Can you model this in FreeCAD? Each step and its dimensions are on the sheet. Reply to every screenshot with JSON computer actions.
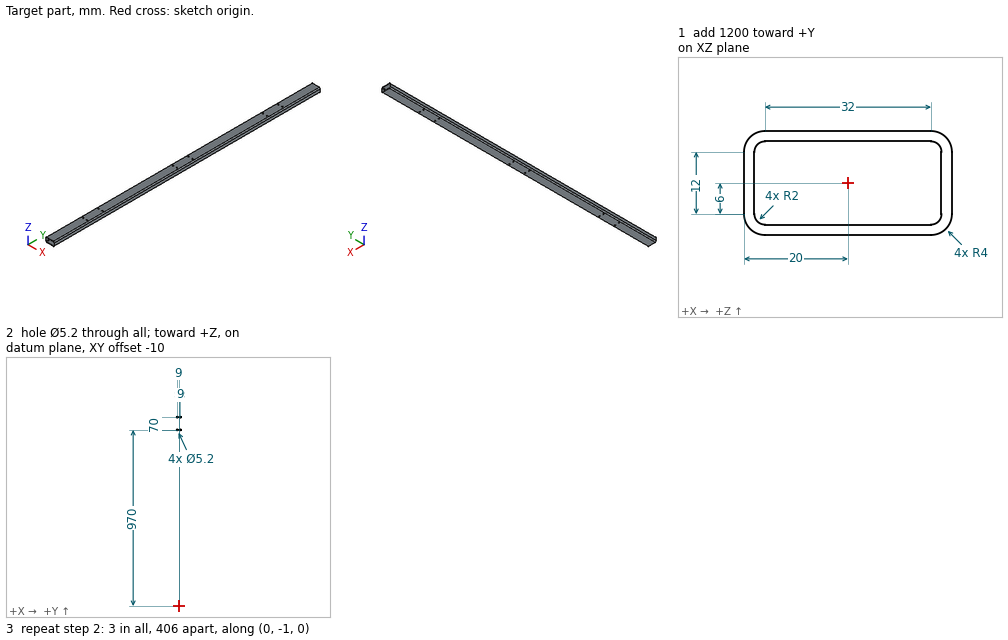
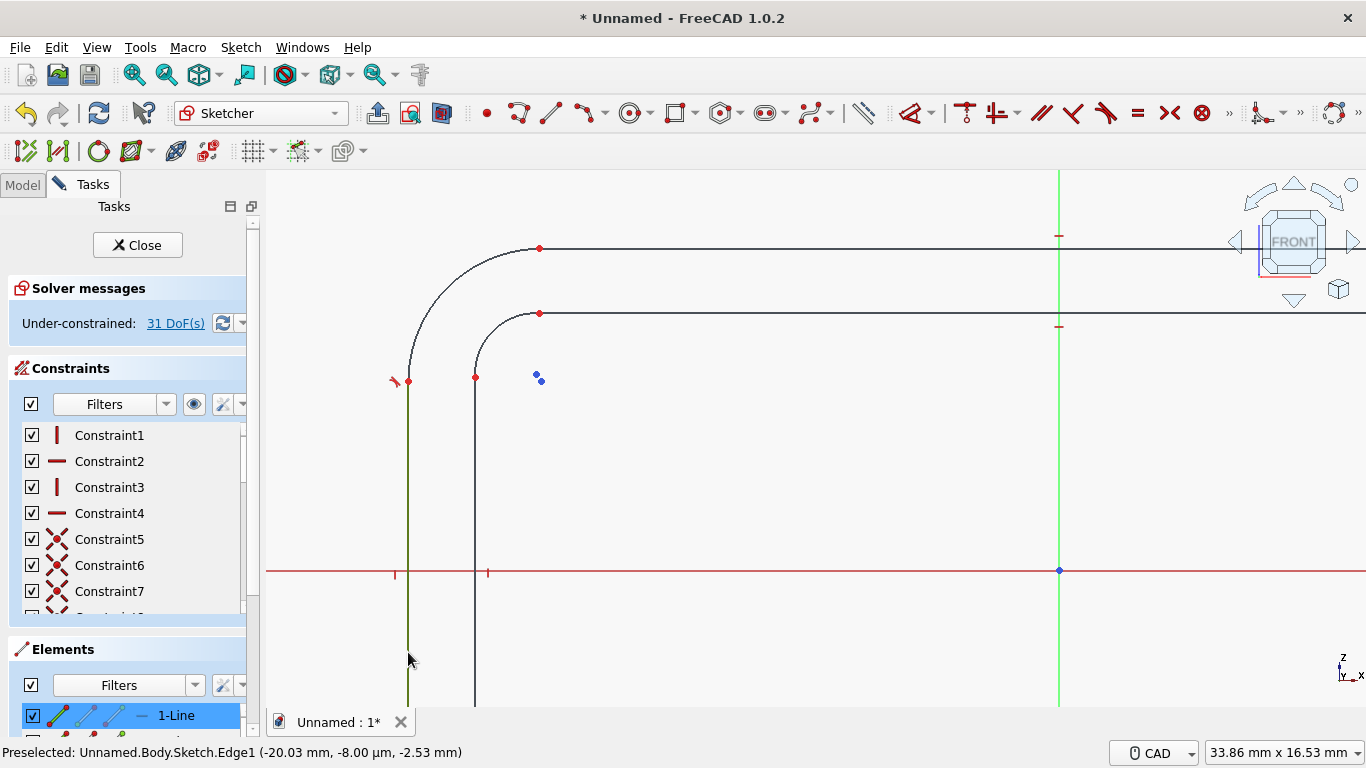
{"action": "scroll", "coordinate": [493, 330], "scroll_direction": "down", "scroll_amount": 4}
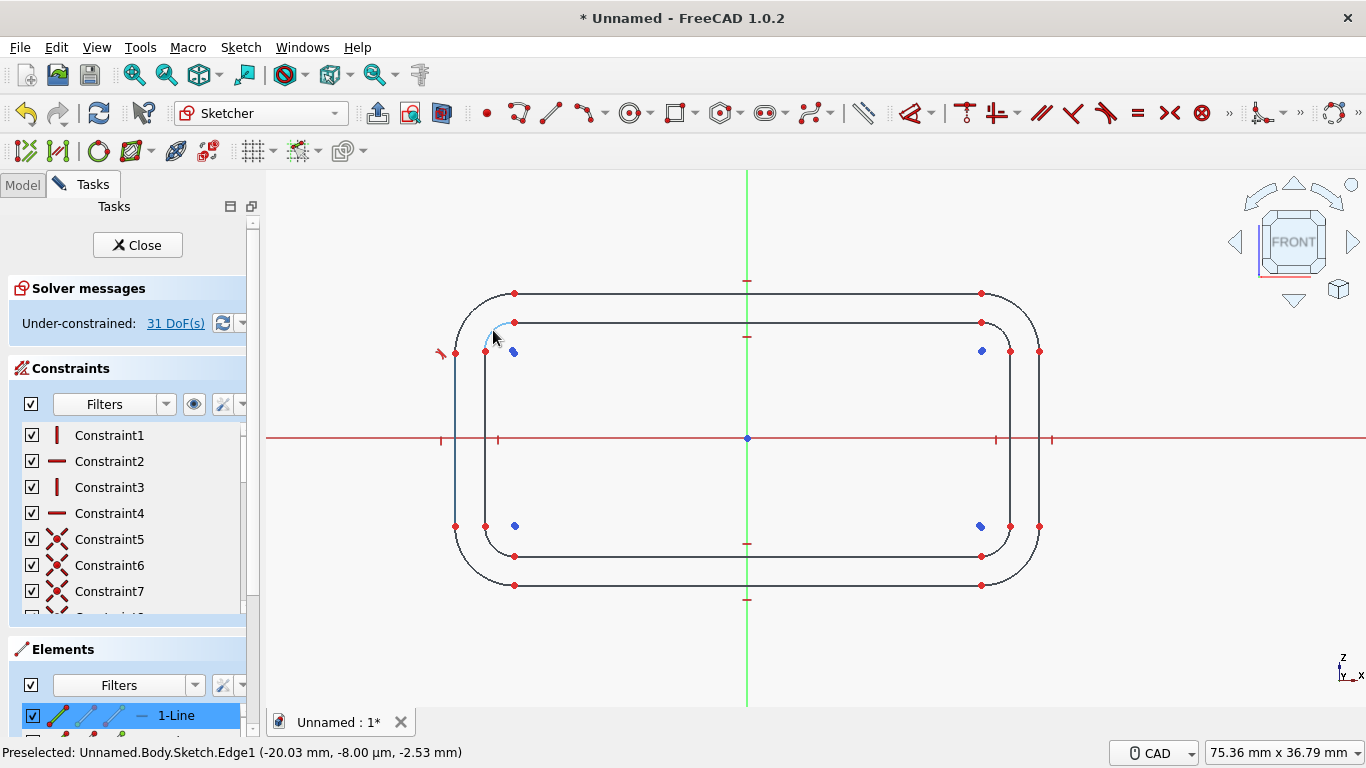
{"action": "left_click", "coordinate": [462, 553]}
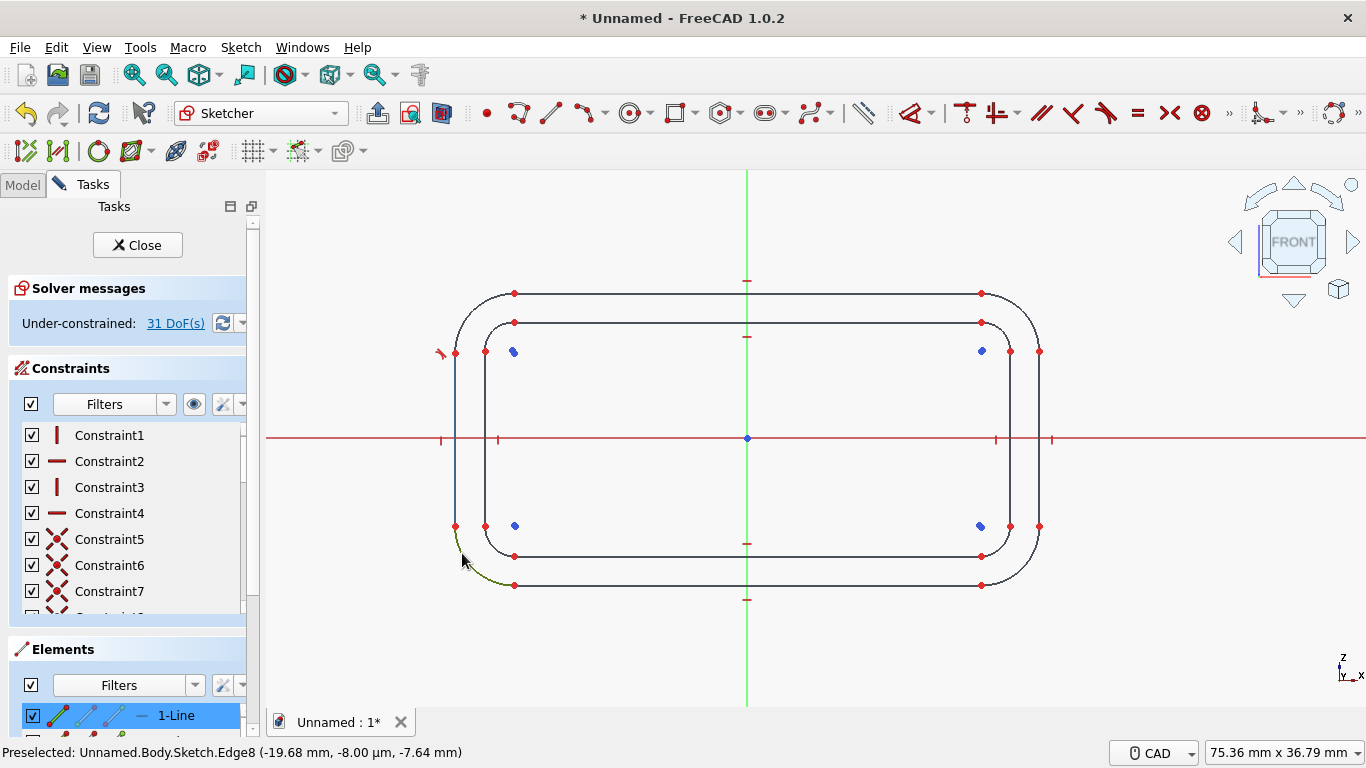
{"action": "left_click", "coordinate": [1106, 114]}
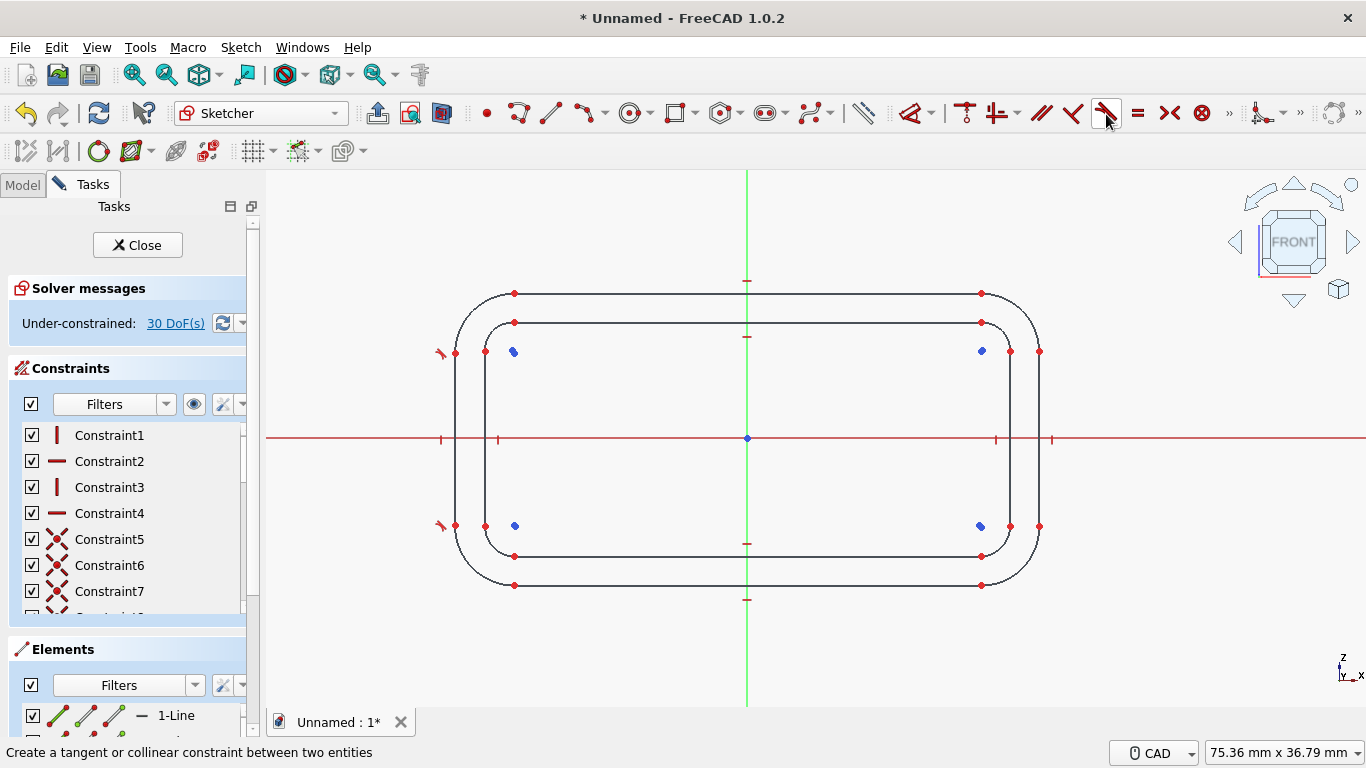
{"action": "left_click", "coordinate": [654, 294]}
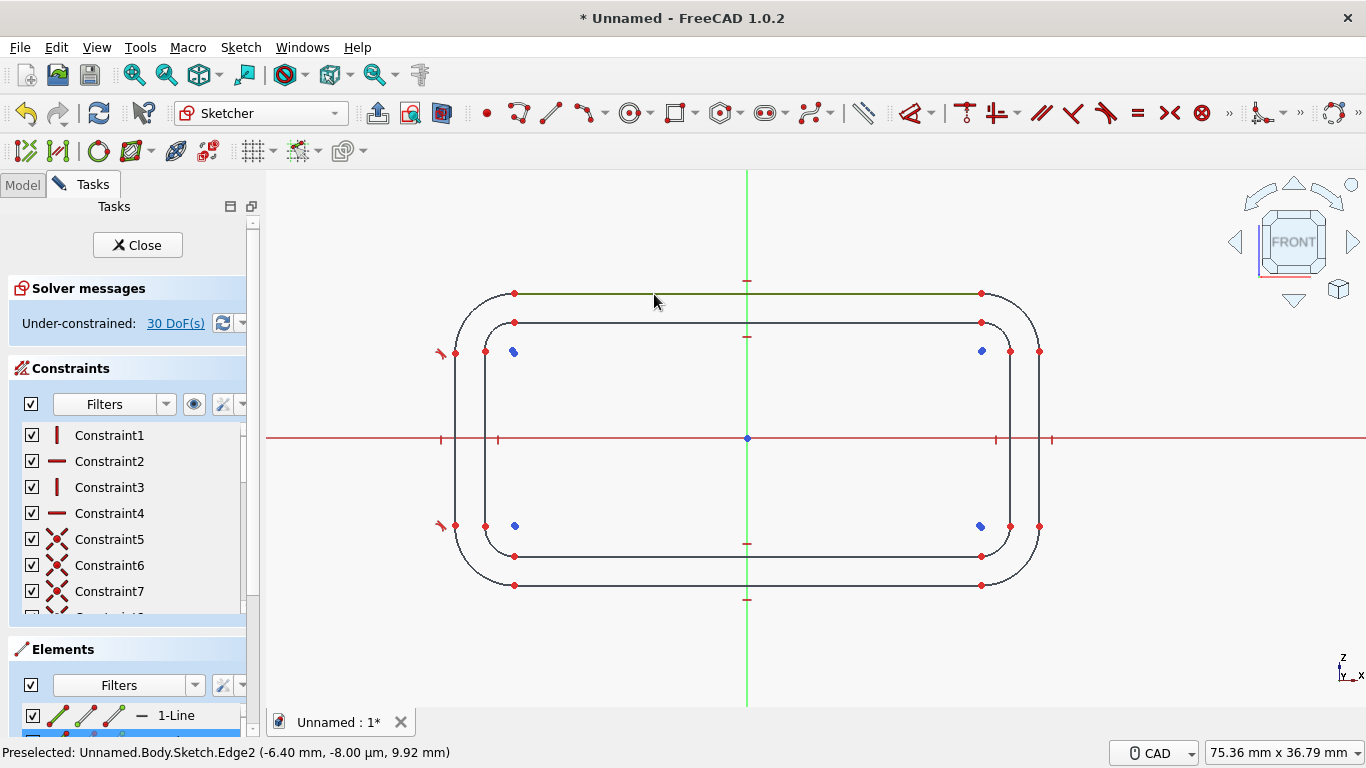
{"action": "left_click", "coordinate": [487, 300]}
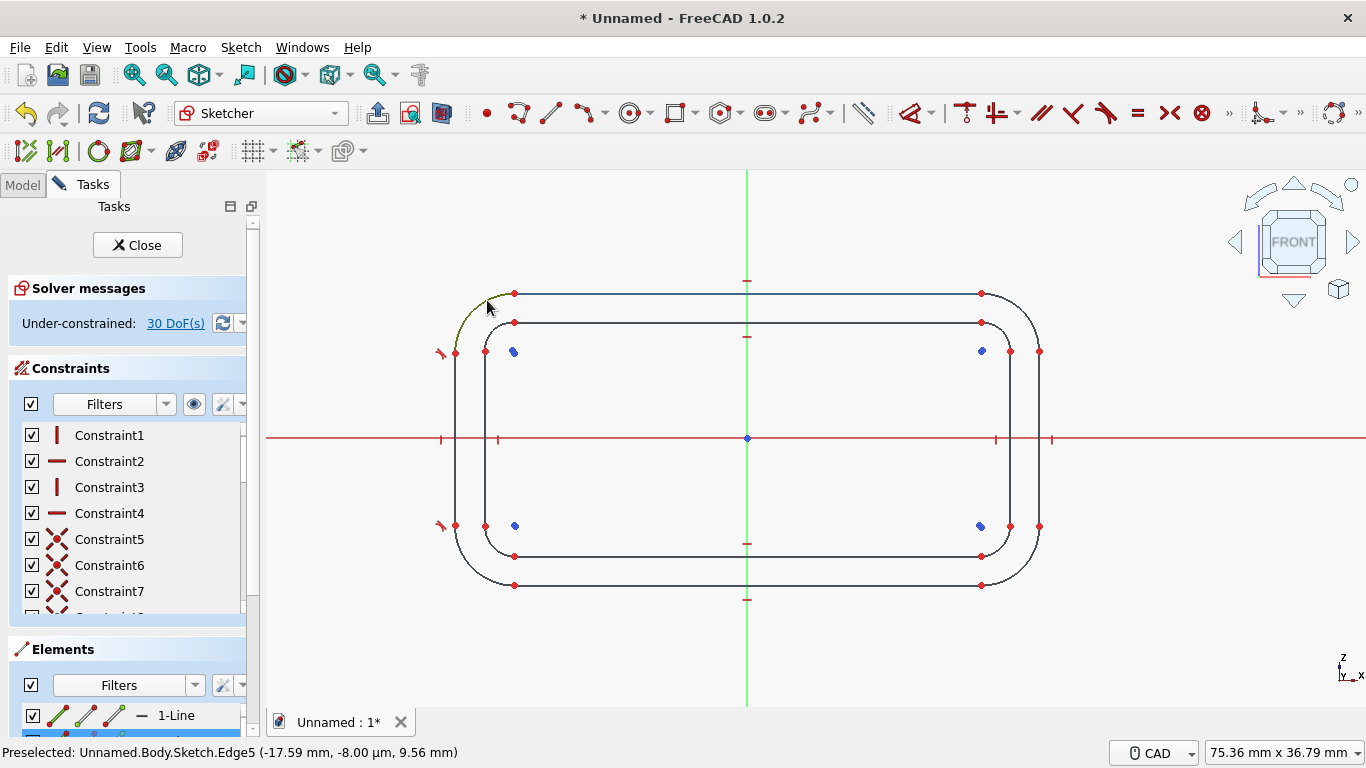
{"action": "left_click", "coordinate": [1106, 114]}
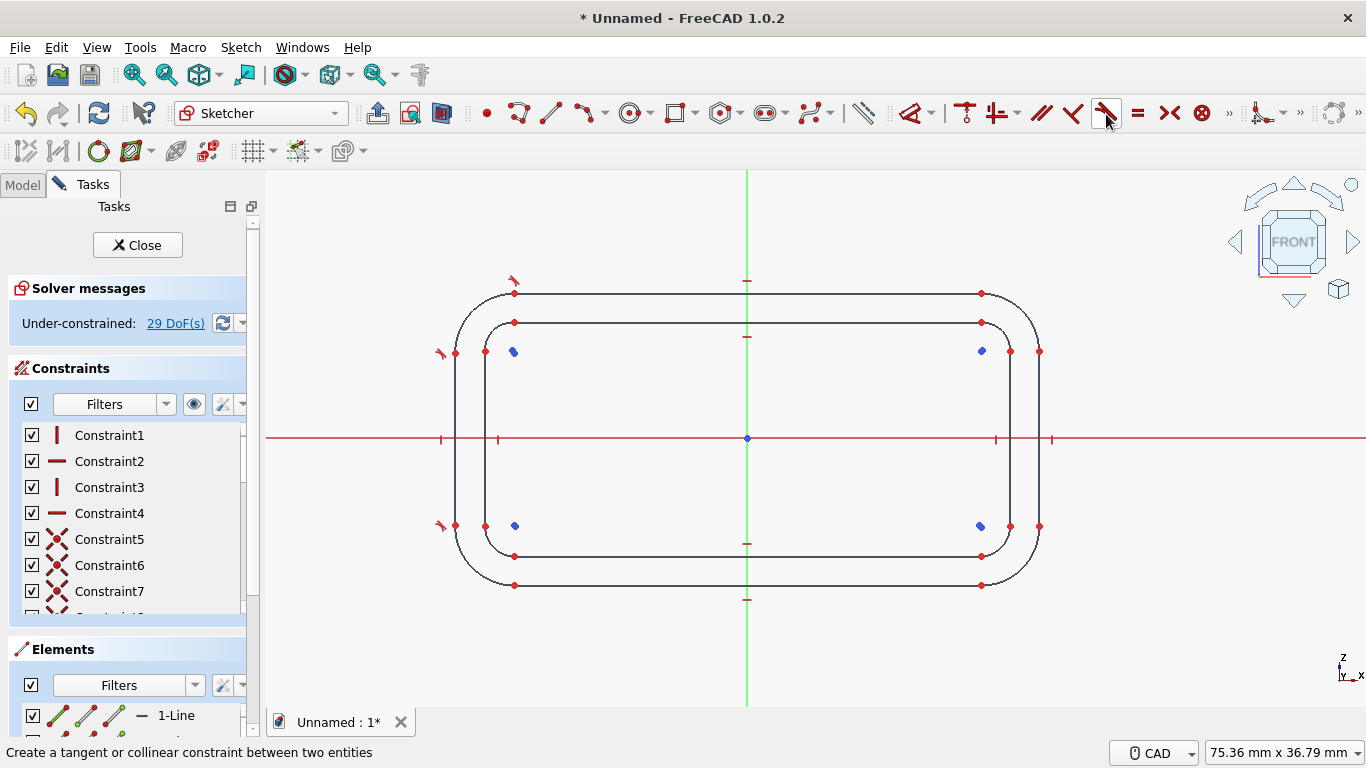
{"action": "left_click", "coordinate": [655, 294]}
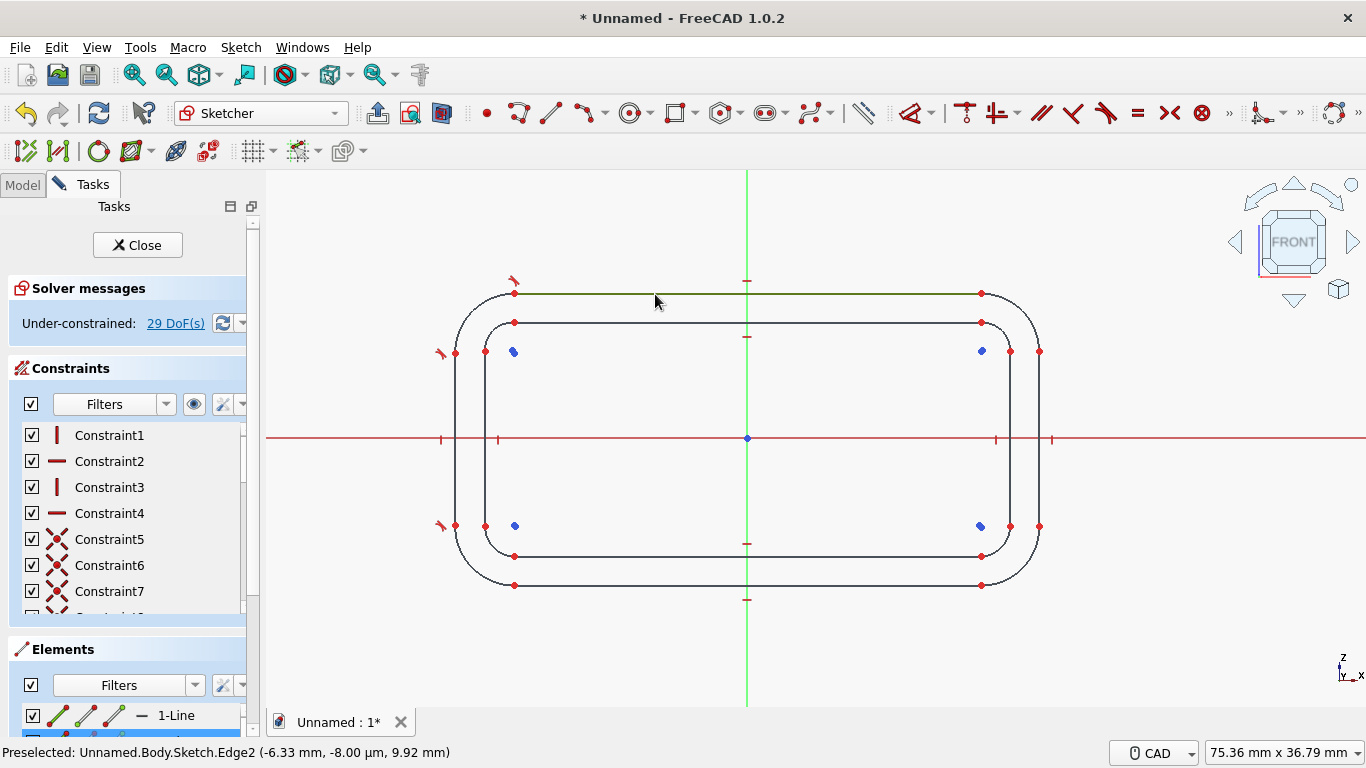
{"action": "left_click", "coordinate": [1033, 325]}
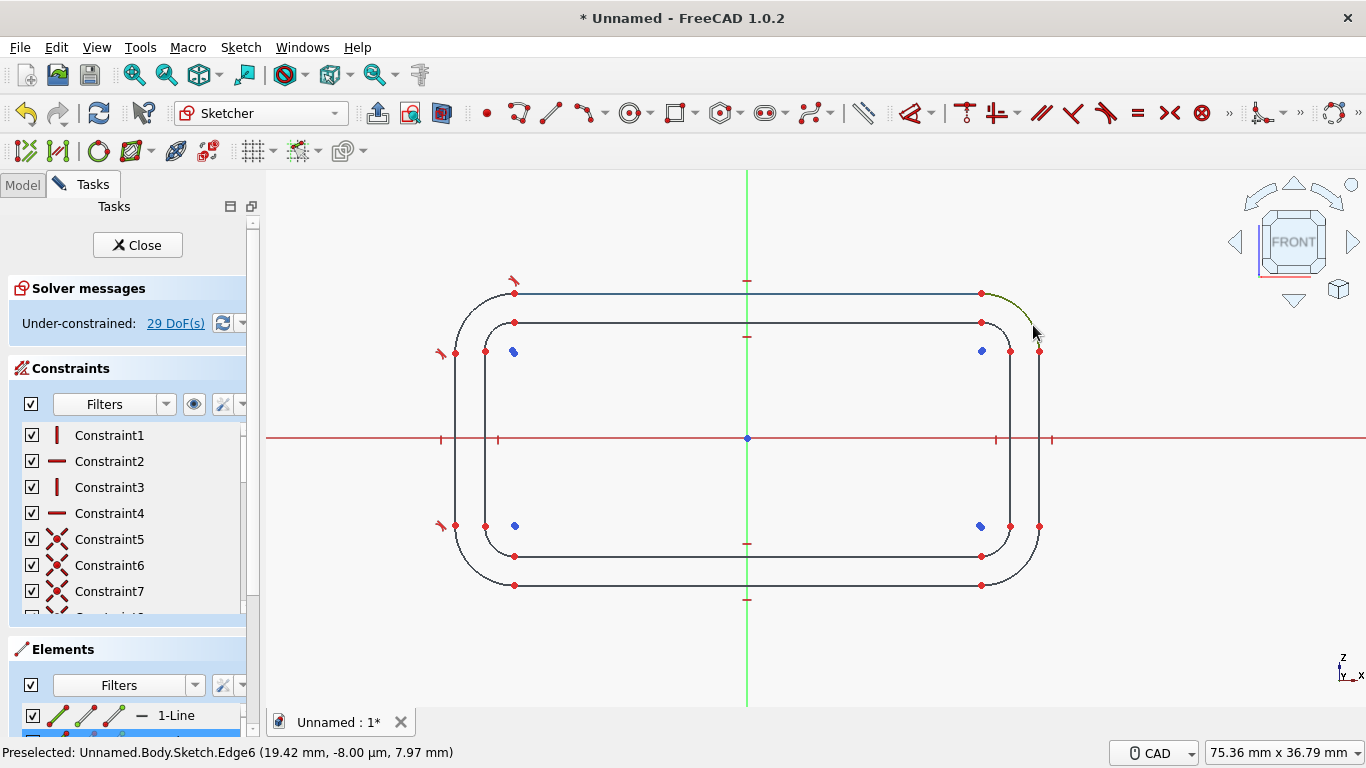
{"action": "left_click", "coordinate": [1106, 114]}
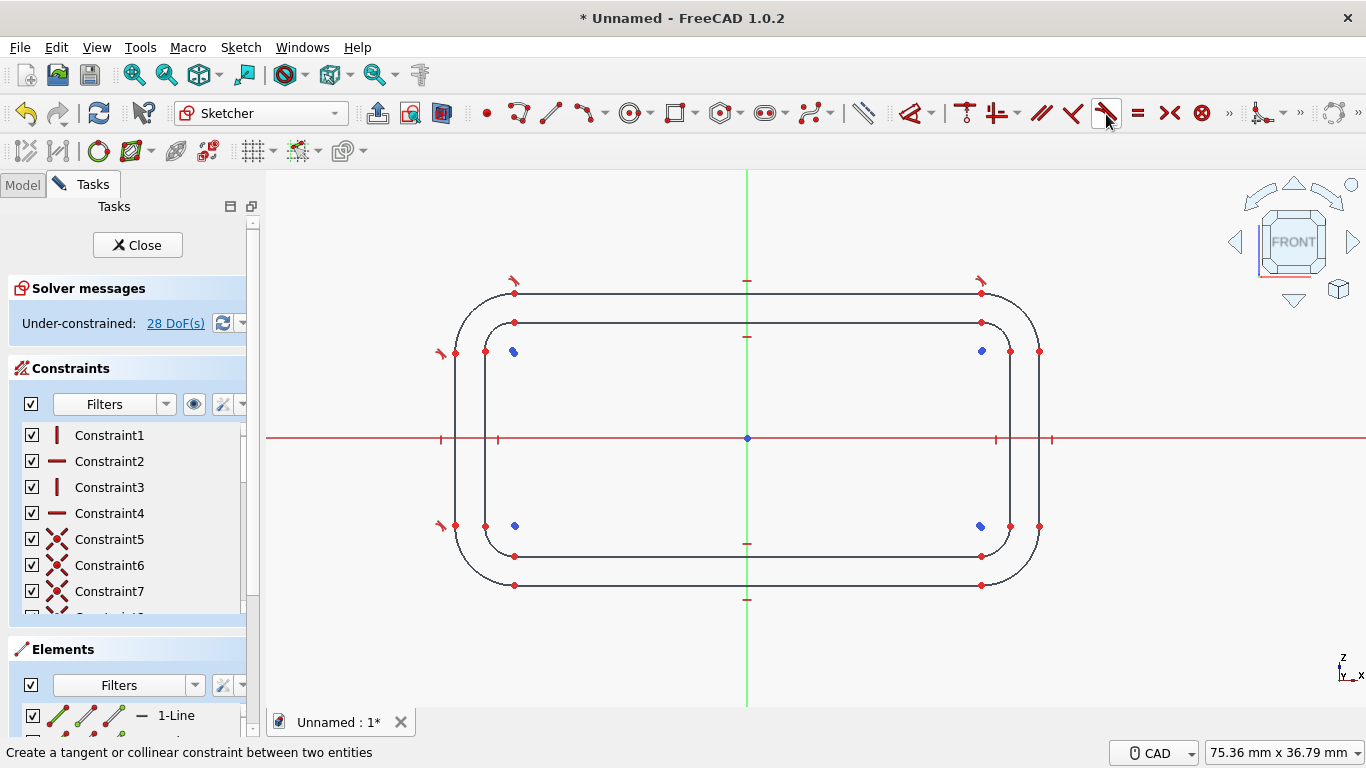
{"action": "left_click", "coordinate": [1039, 404]}